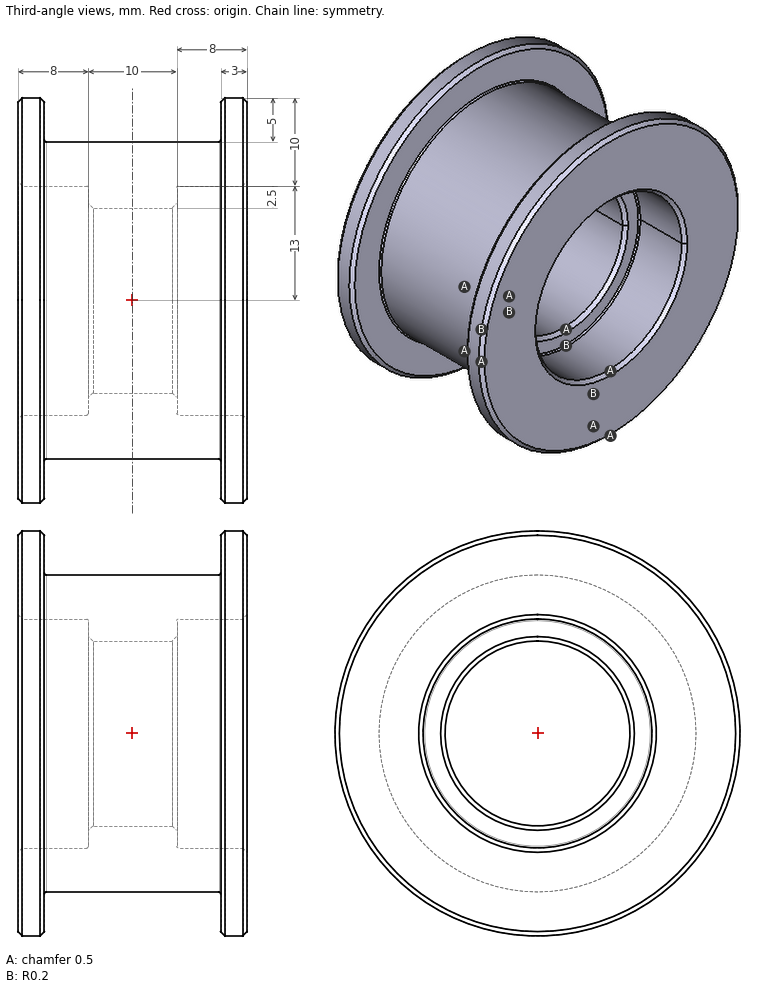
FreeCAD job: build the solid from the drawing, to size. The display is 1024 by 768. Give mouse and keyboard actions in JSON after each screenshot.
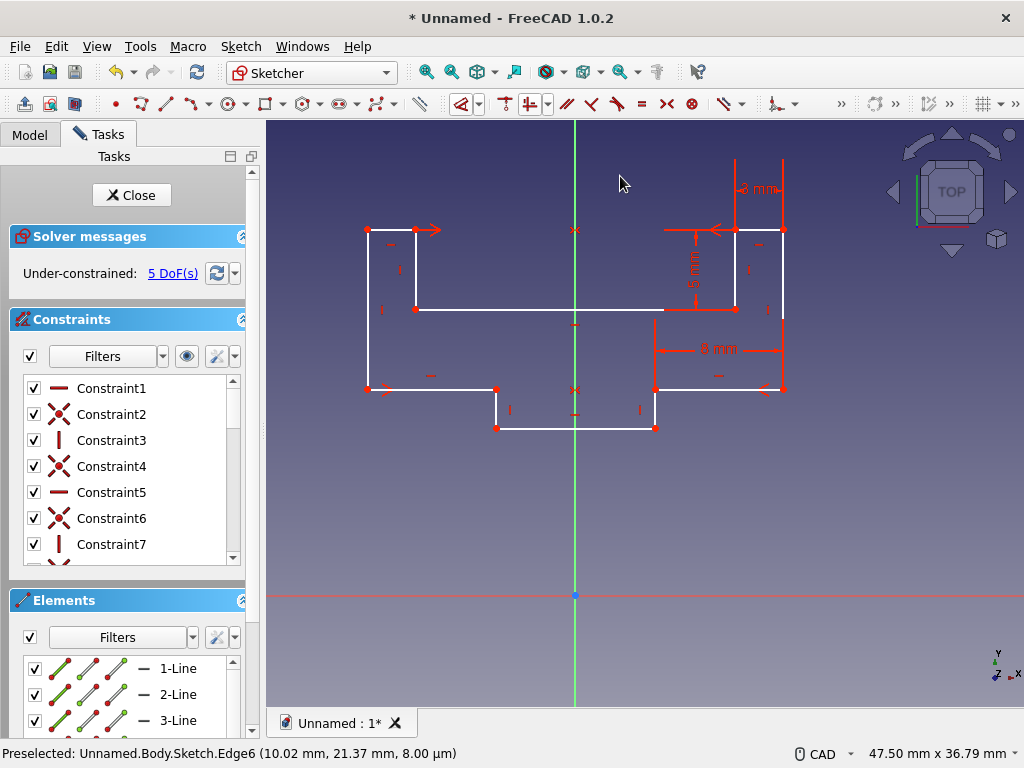
{"action": "left_click", "coordinate": [406, 390]}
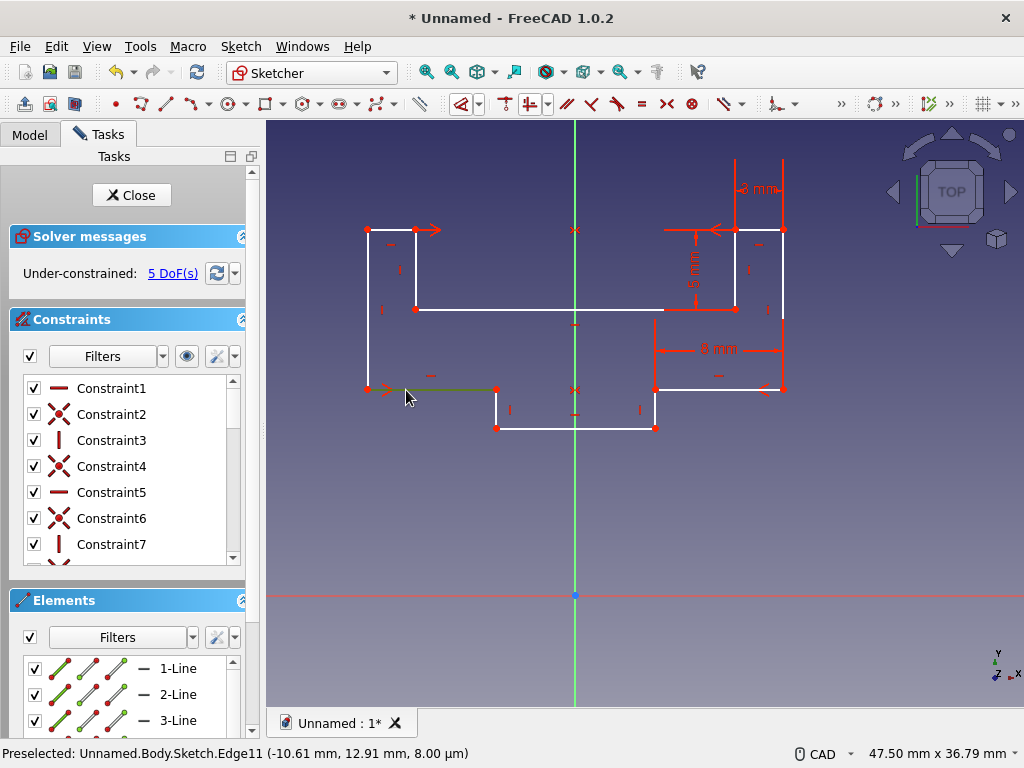
{"action": "key", "text": "l"}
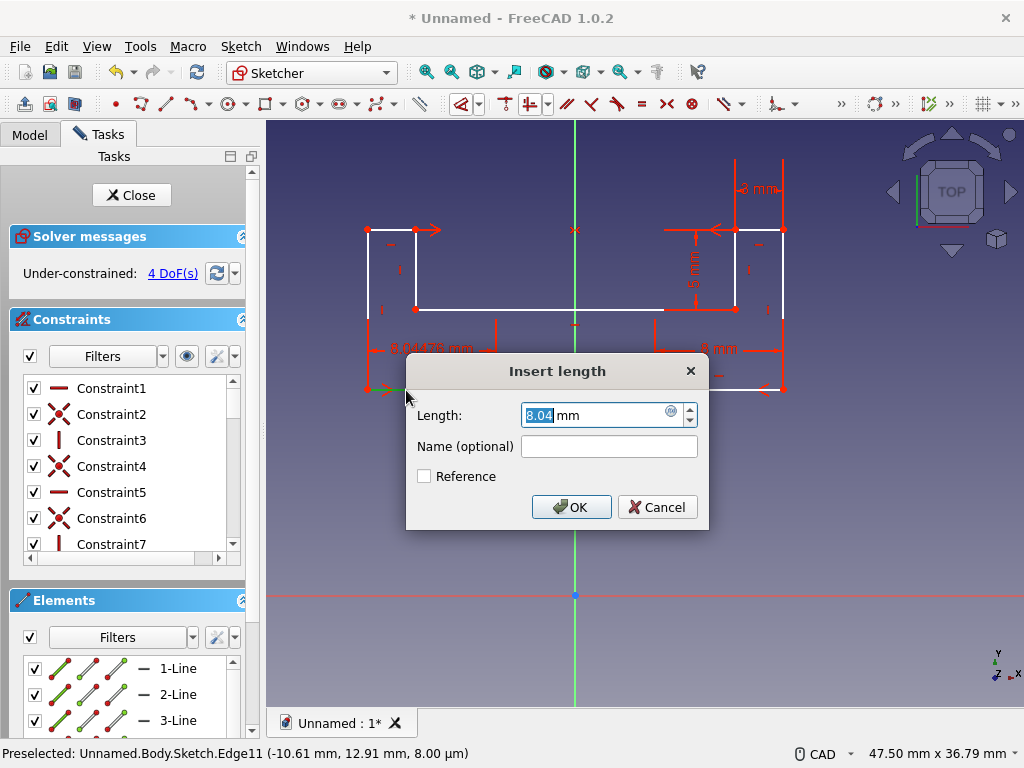
{"action": "type", "text": "8"}
{"action": "key", "text": "Return"}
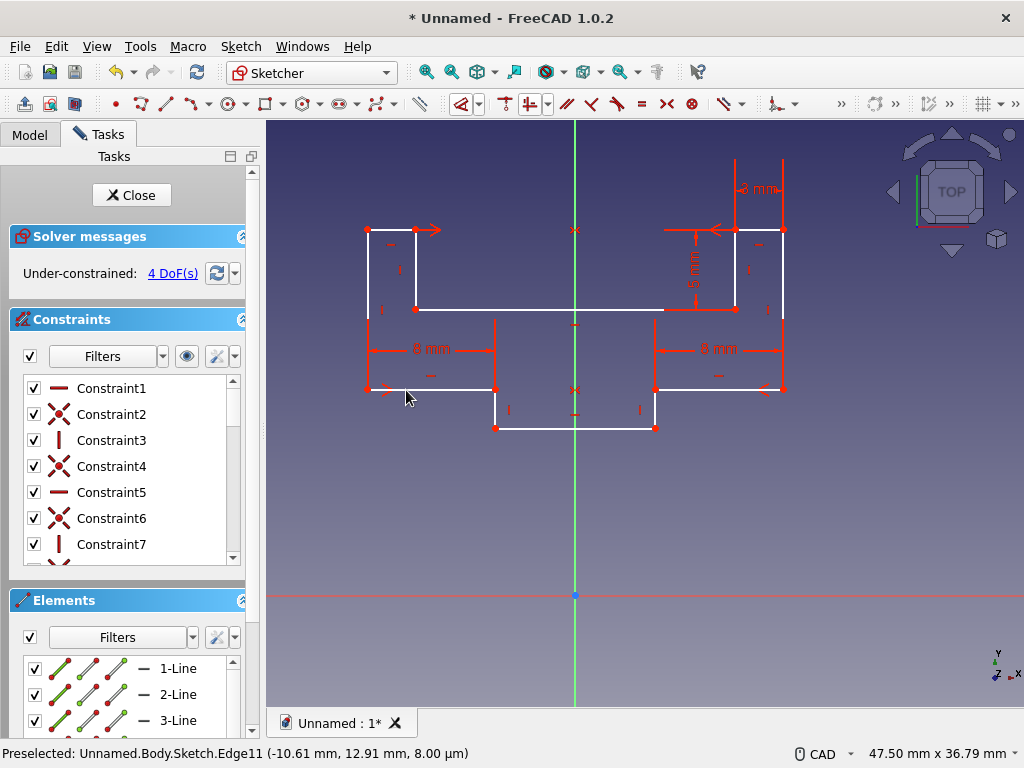
{"action": "left_click", "coordinate": [543, 429]}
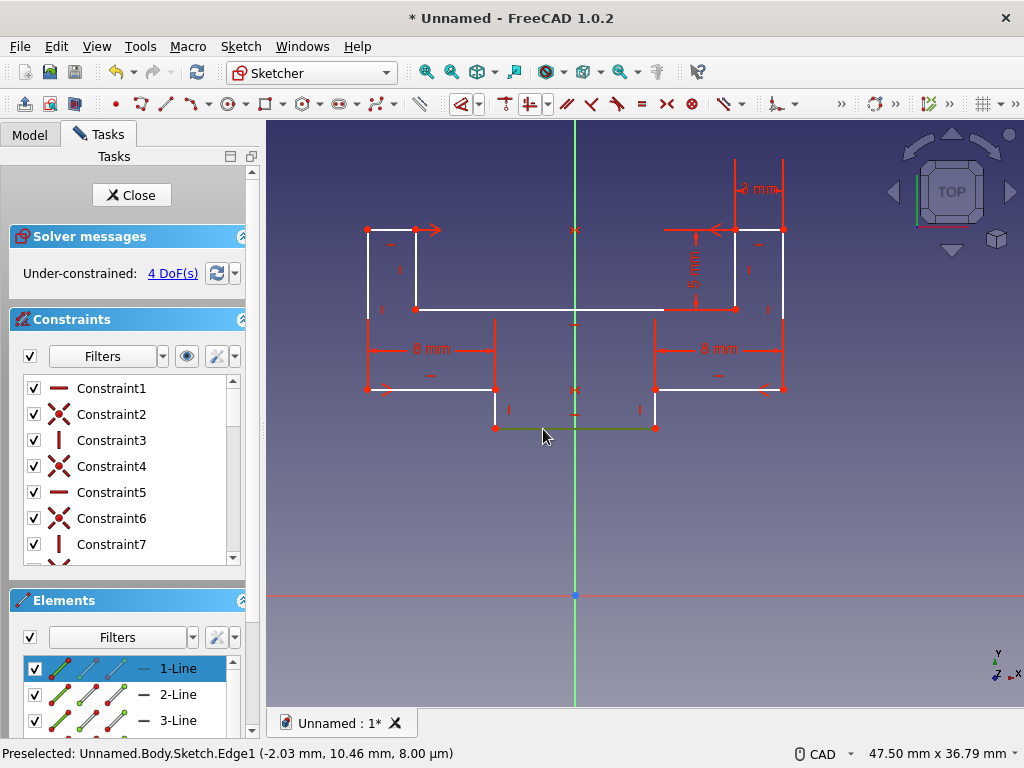
{"action": "key", "text": "l"}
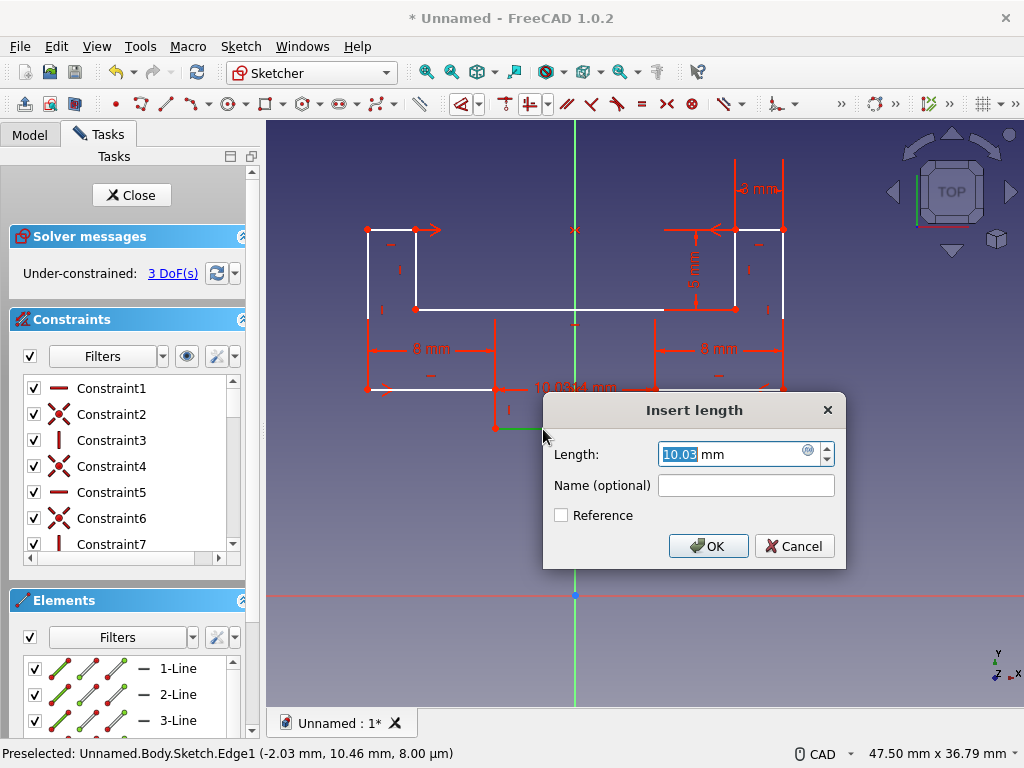
{"action": "type", "text": "10"}
{"action": "key", "text": "Return"}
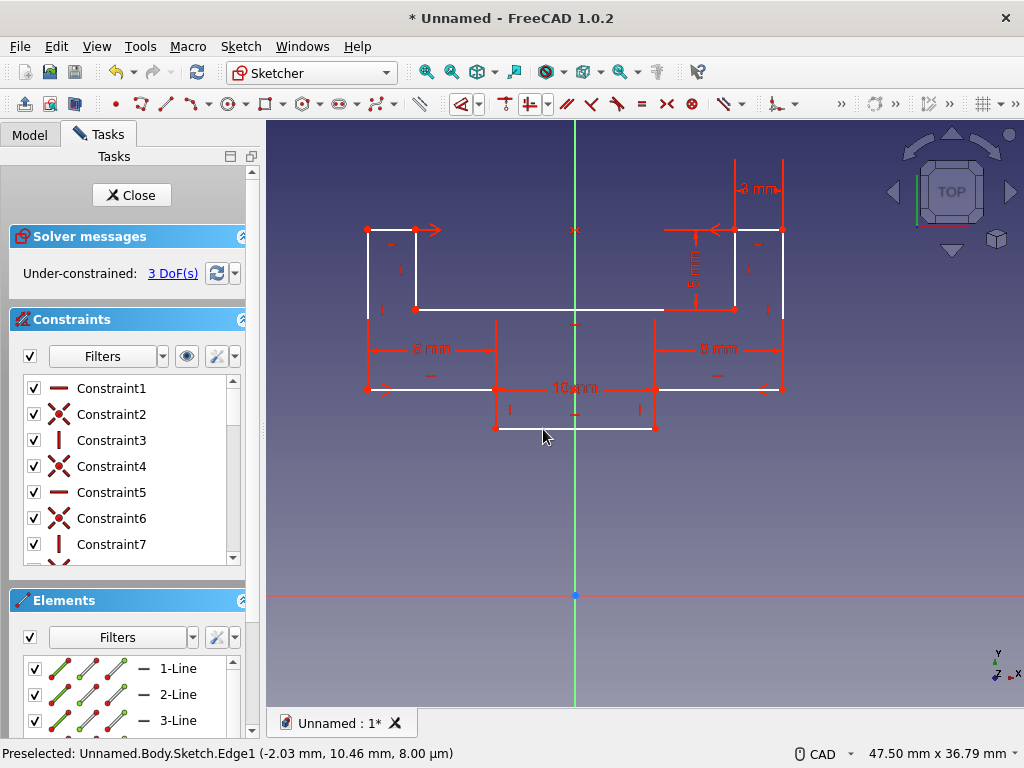
{"action": "left_click", "coordinate": [783, 342]}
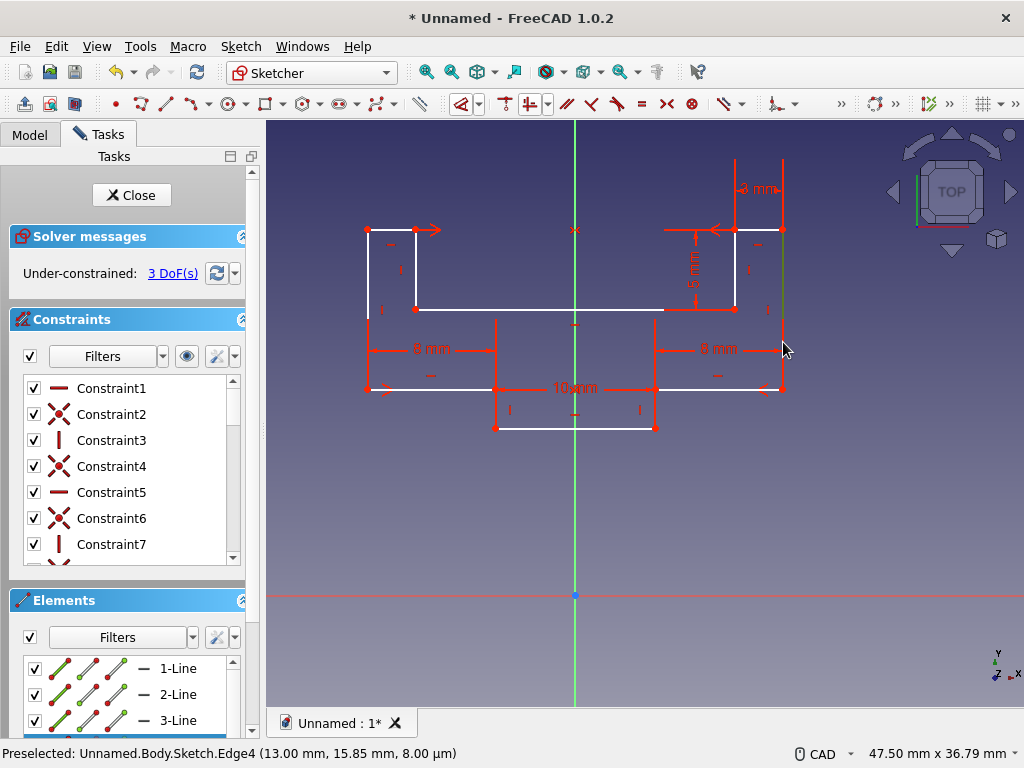
{"action": "left_click", "coordinate": [478, 104]}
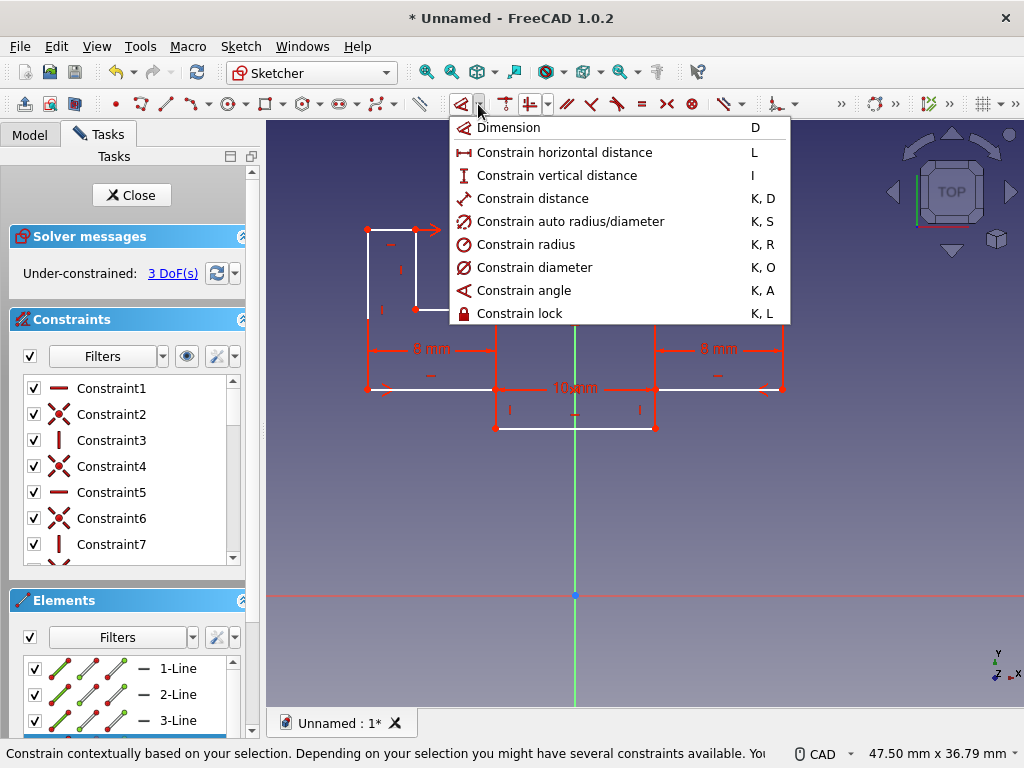
{"action": "left_click", "coordinate": [620, 176]}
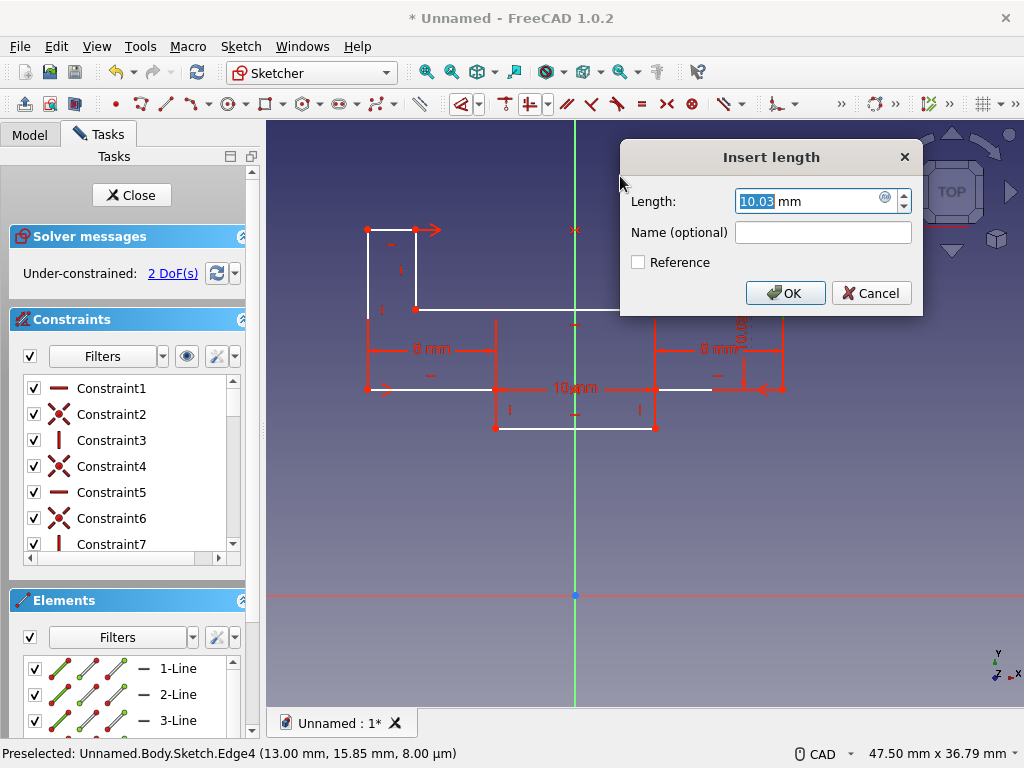
{"action": "type", "text": "10"}
{"action": "key", "text": "Return"}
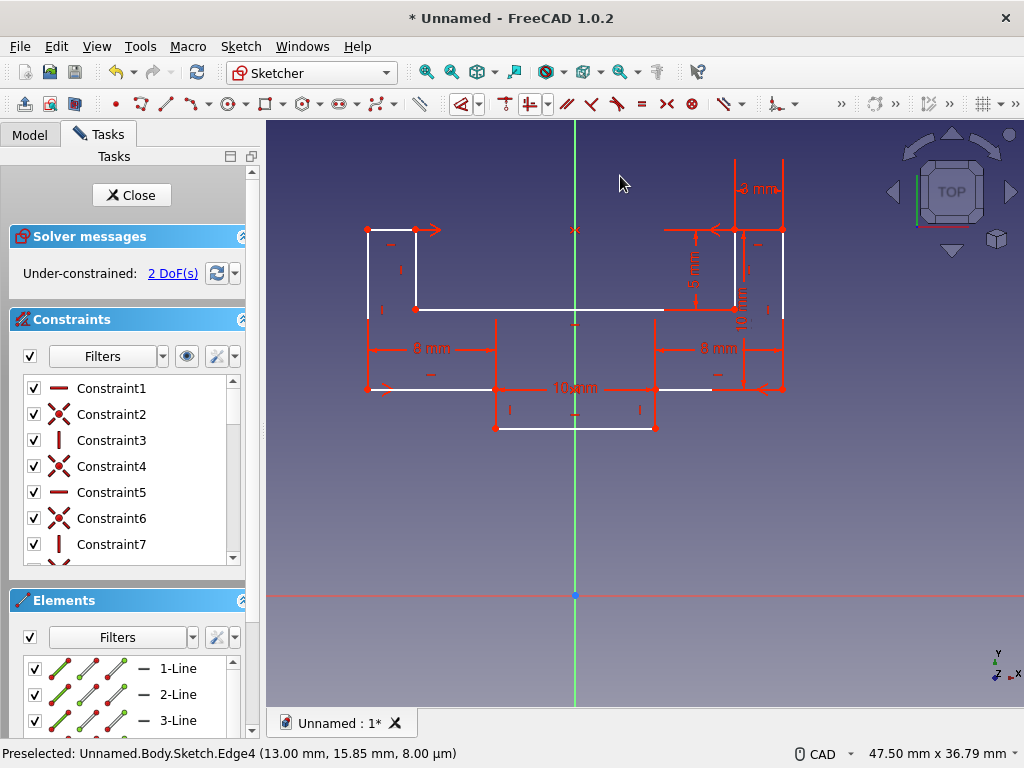
{"action": "left_click", "coordinate": [655, 417]}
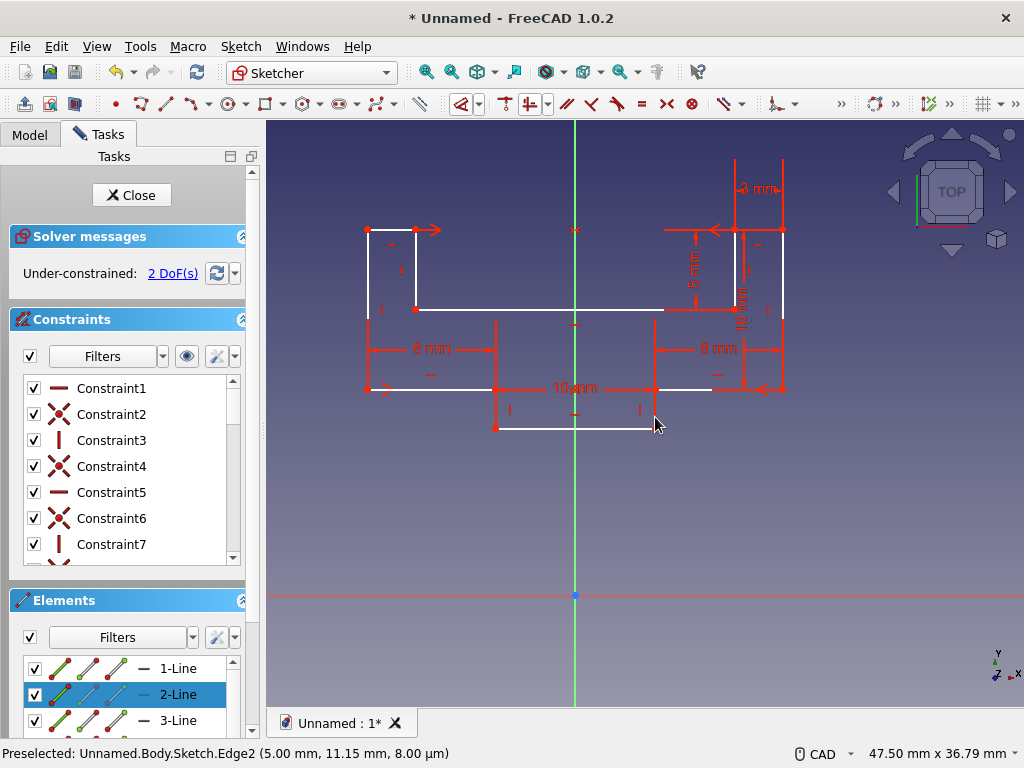
{"action": "key", "text": "i"}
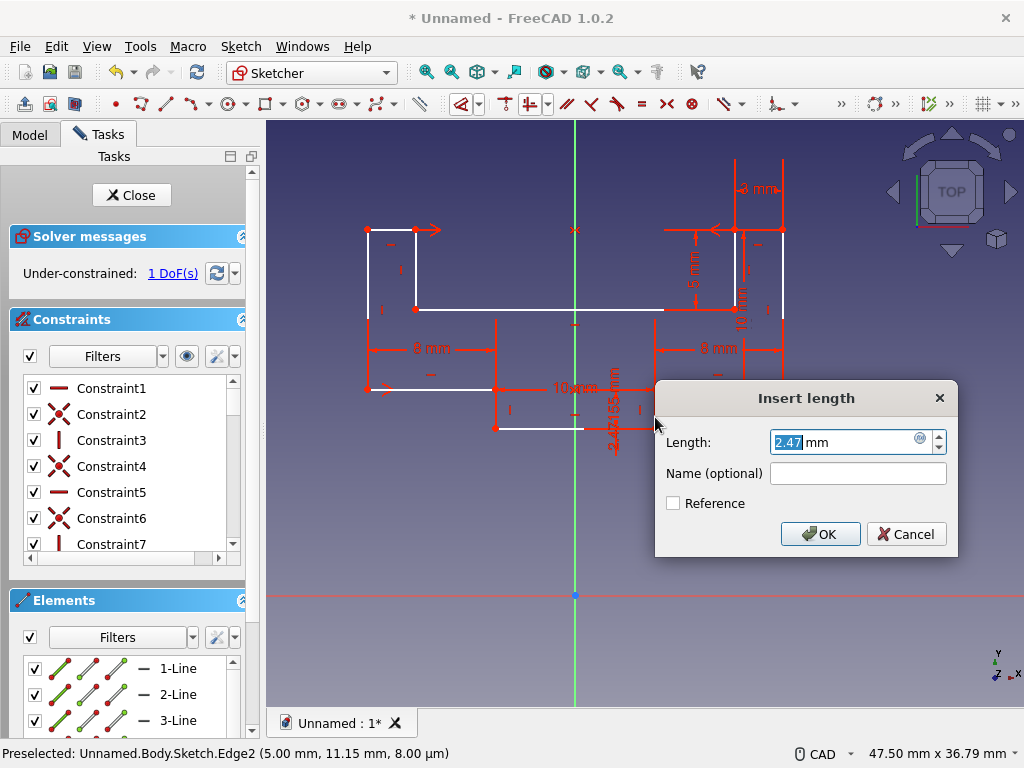
{"action": "type", "text": "2.5"}
{"action": "key", "text": "Return"}